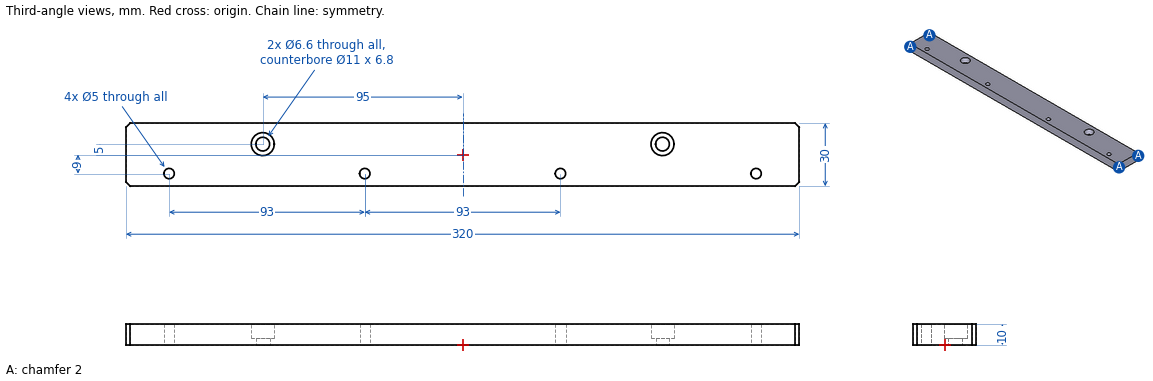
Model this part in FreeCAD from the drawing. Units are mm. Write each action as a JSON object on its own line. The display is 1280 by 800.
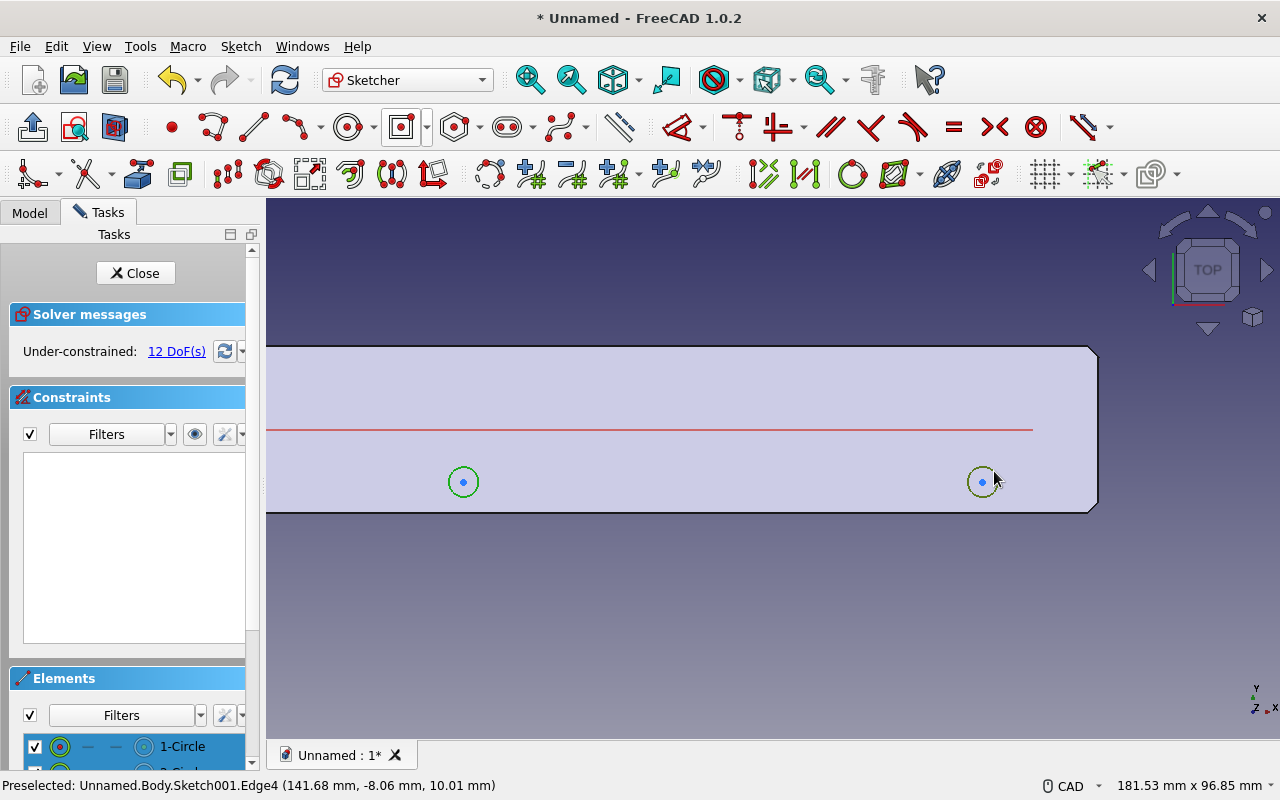
{"action": "left_click", "coordinate": [954, 128]}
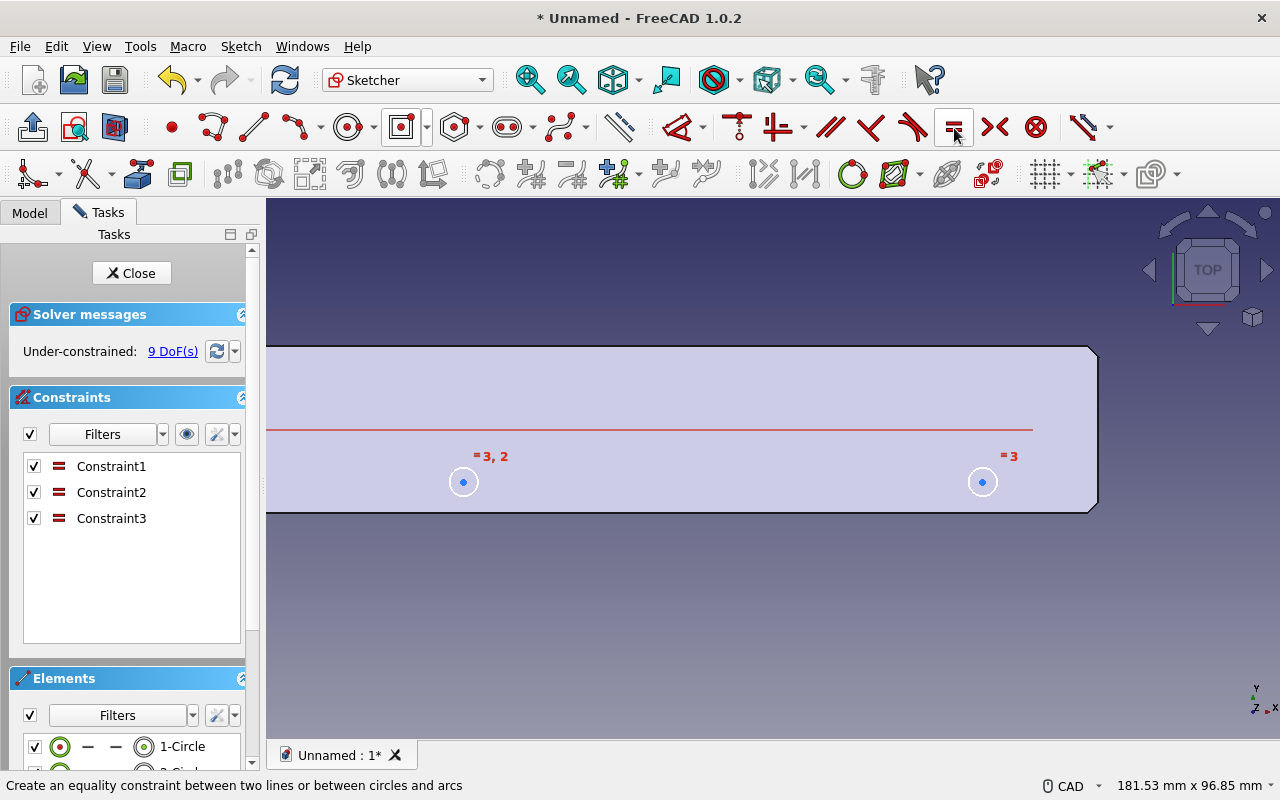
{"action": "scroll", "coordinate": [995, 472], "scroll_direction": "down", "scroll_amount": 5}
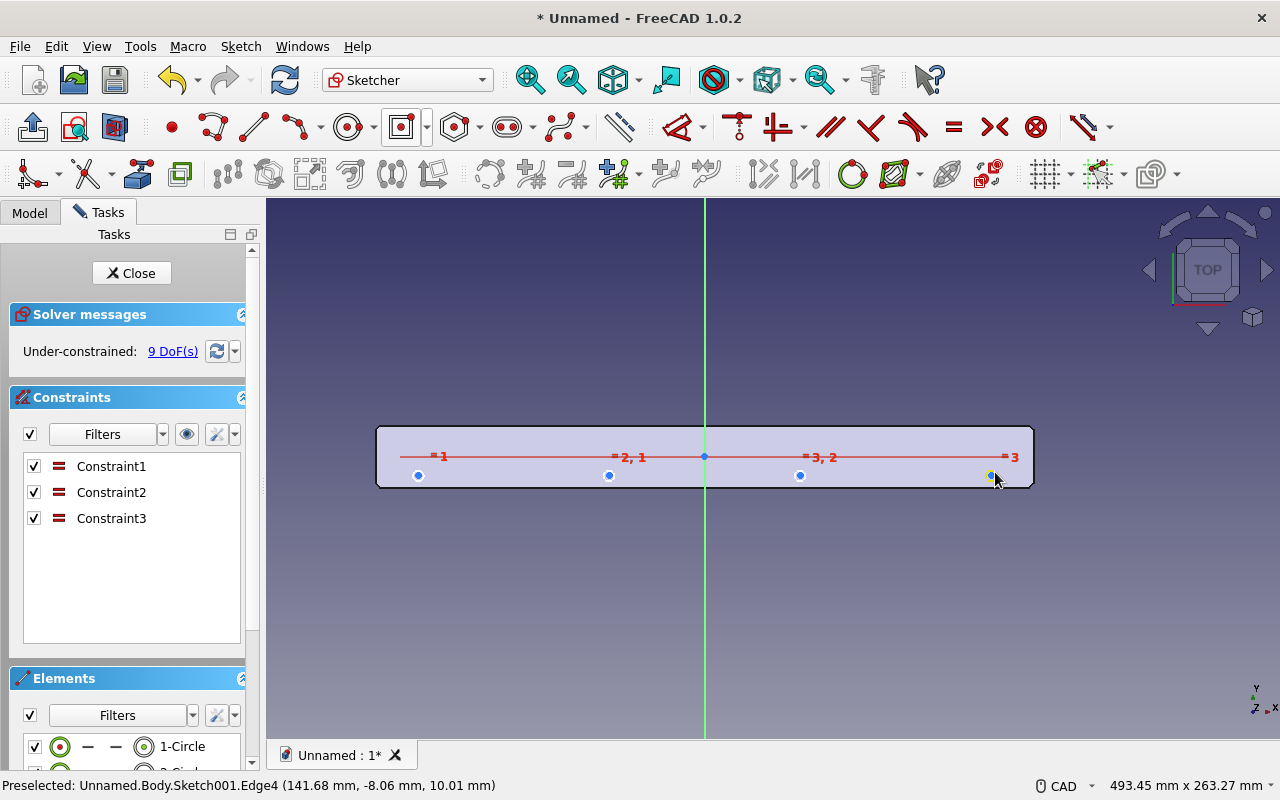
{"action": "left_click", "coordinate": [609, 476]}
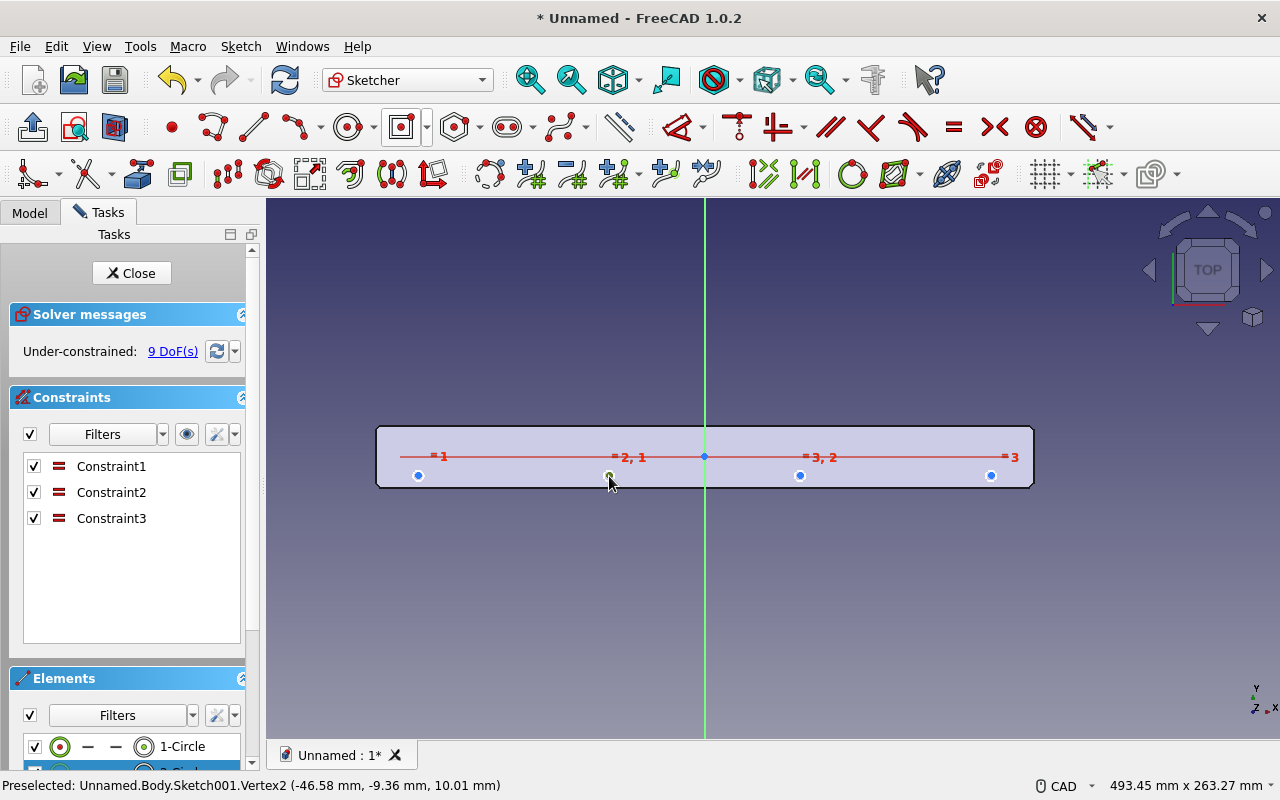
{"action": "left_click", "coordinate": [800, 476]}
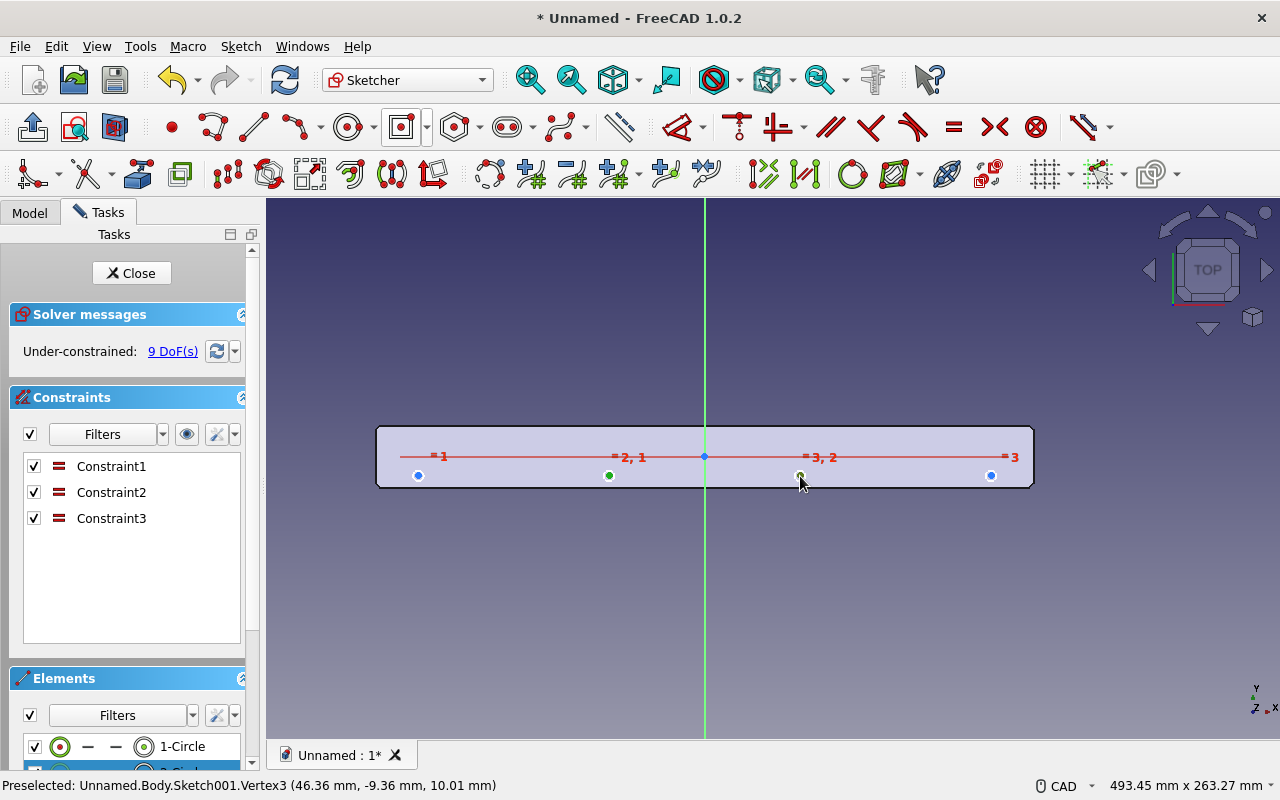
{"action": "left_click", "coordinate": [705, 676]}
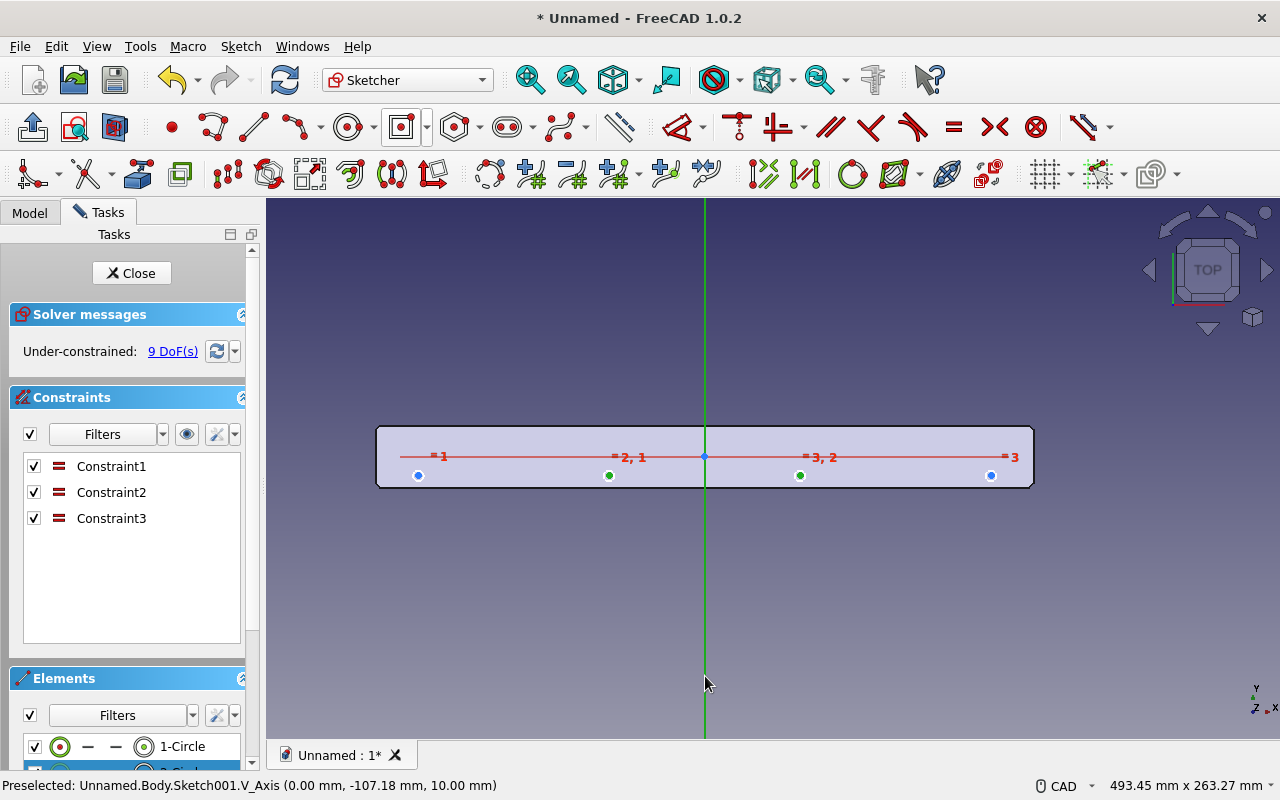
{"action": "left_click", "coordinate": [995, 128]}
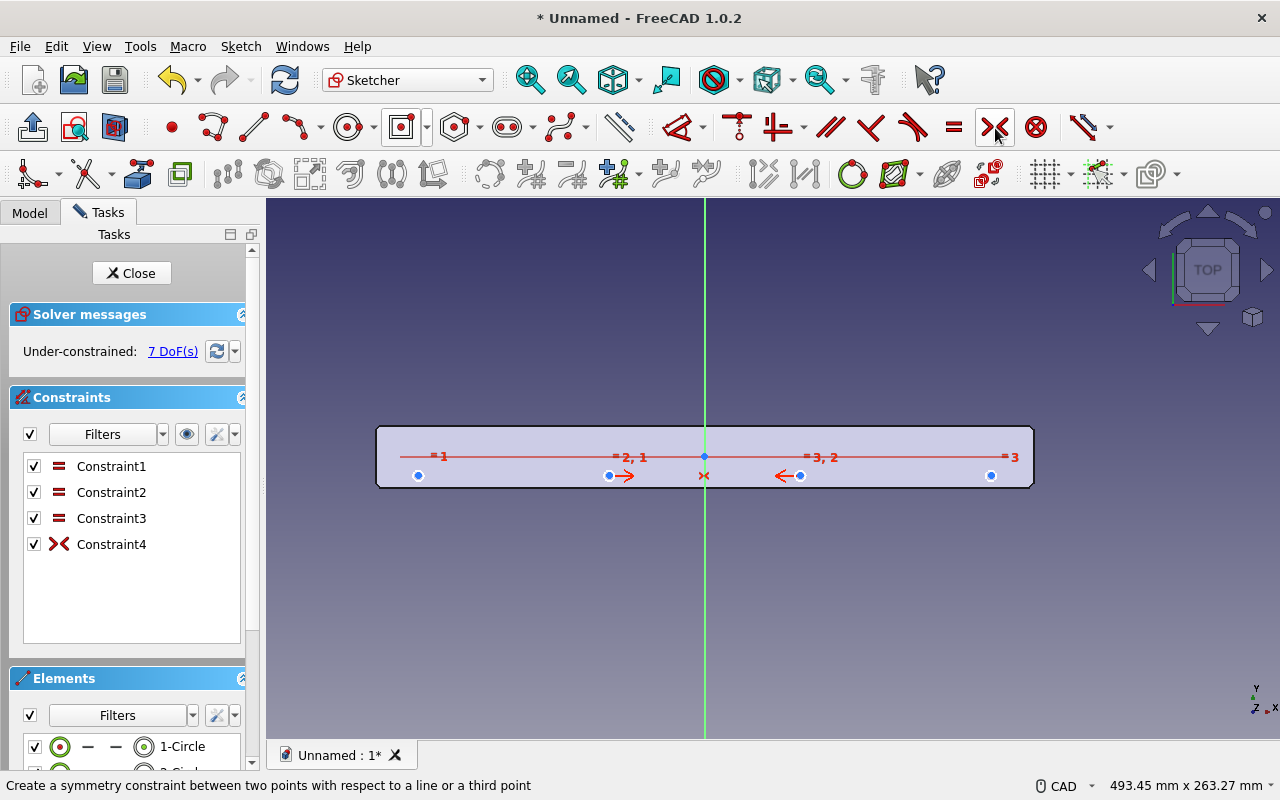
{"action": "left_click", "coordinate": [418, 476]}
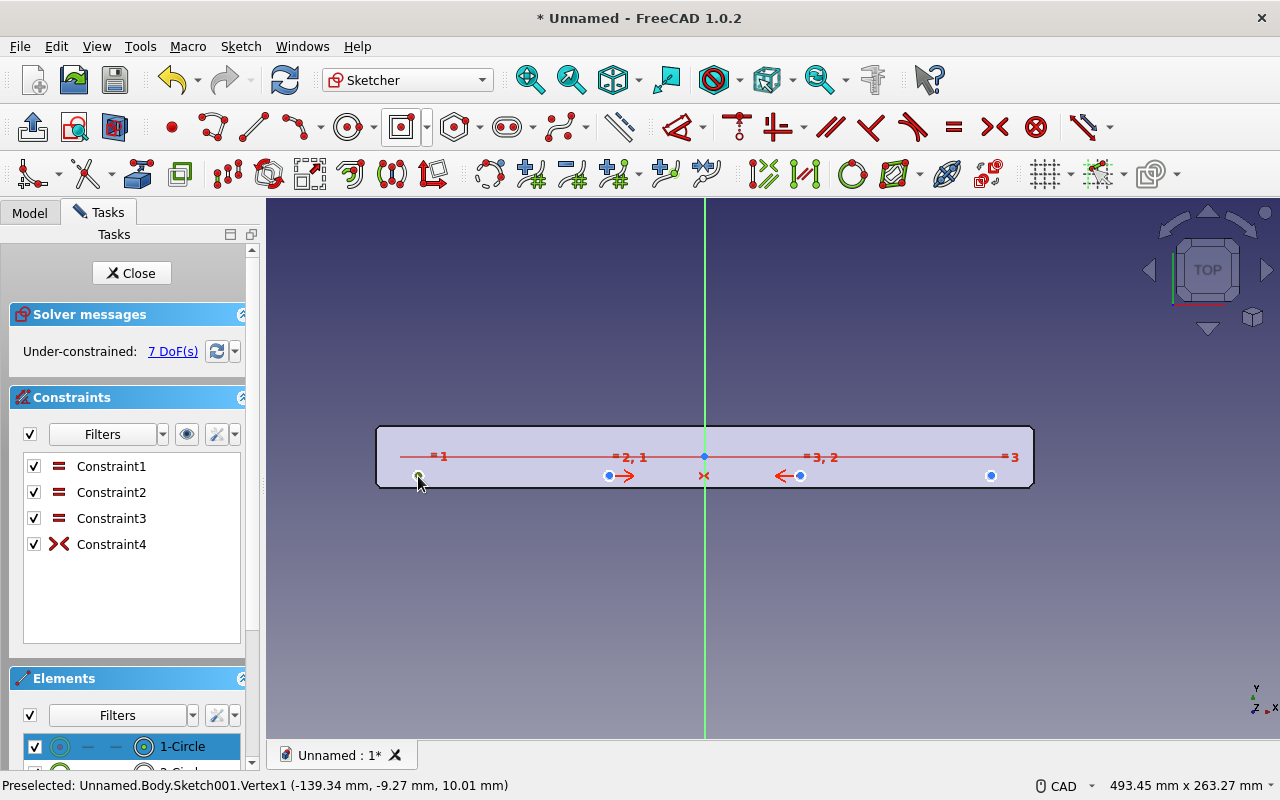
{"action": "left_click", "coordinate": [991, 476]}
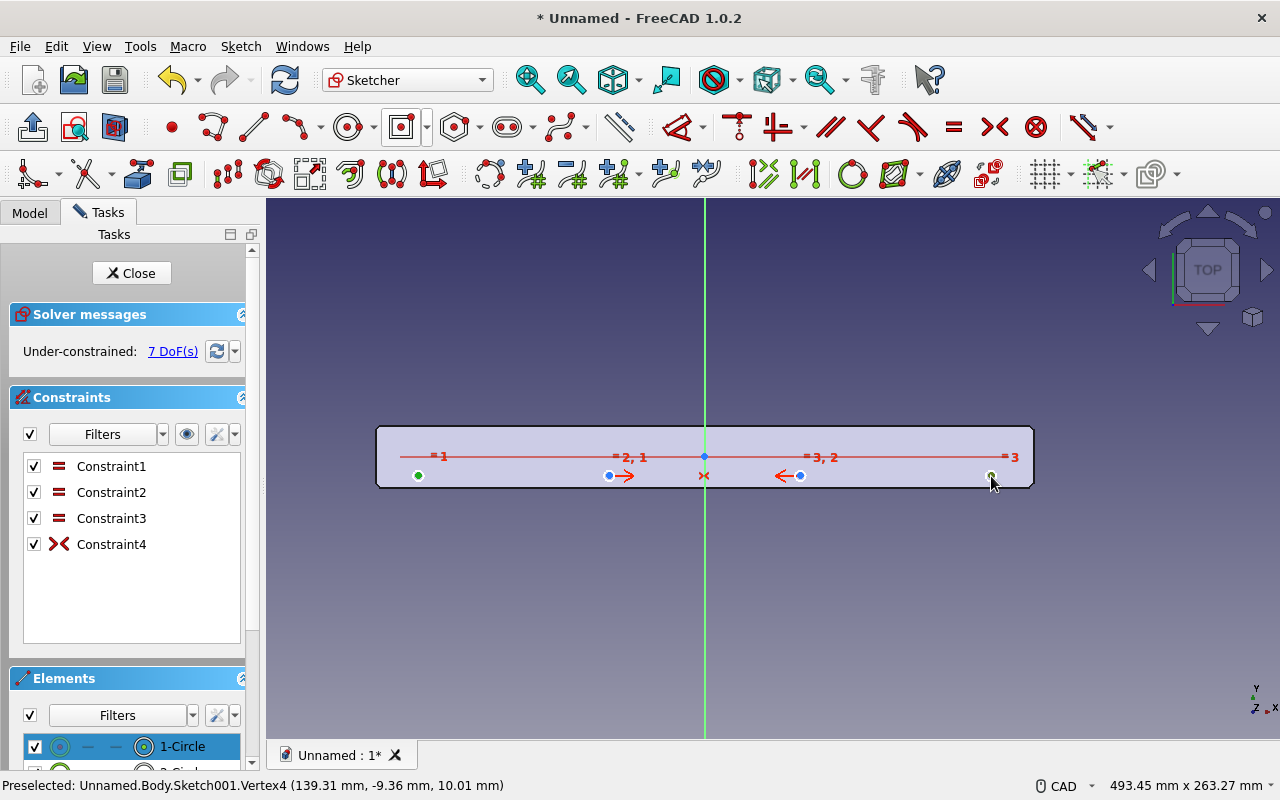
{"action": "left_click", "coordinate": [705, 676]}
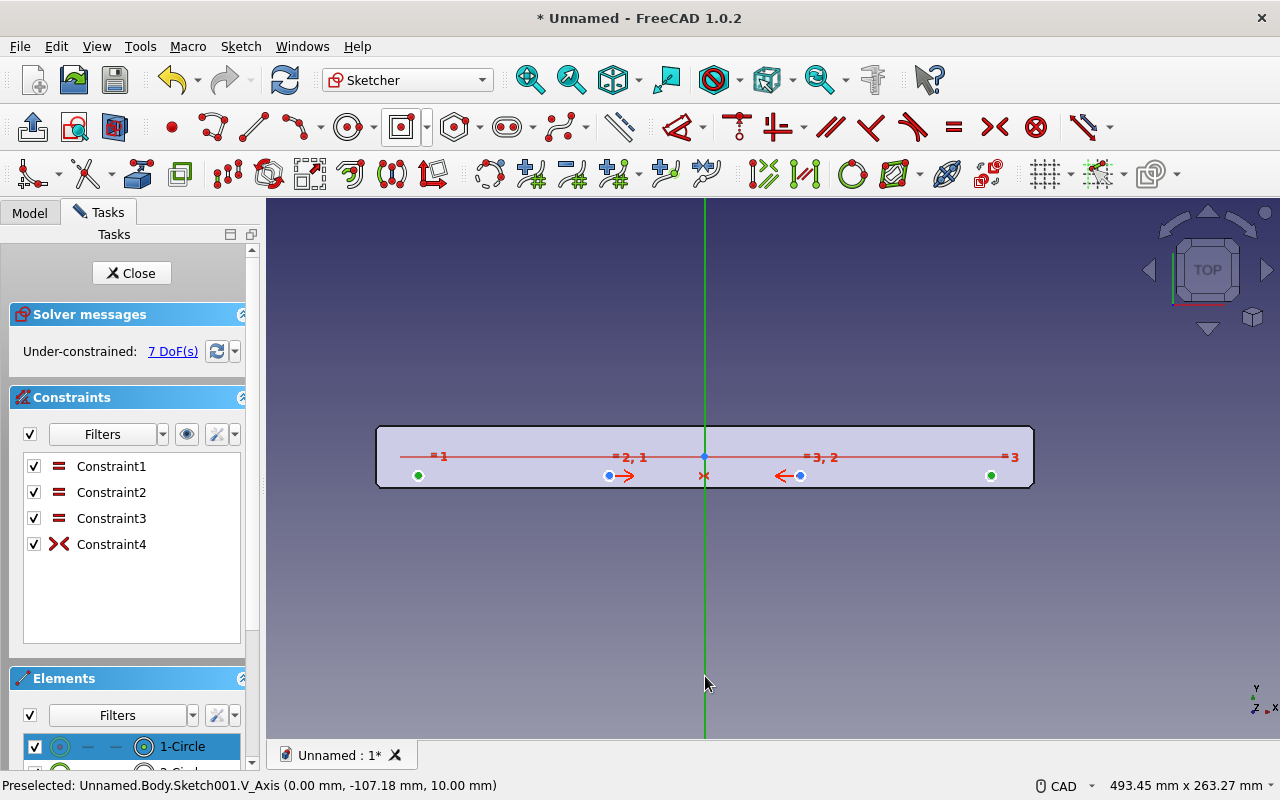
{"action": "left_click", "coordinate": [995, 128]}